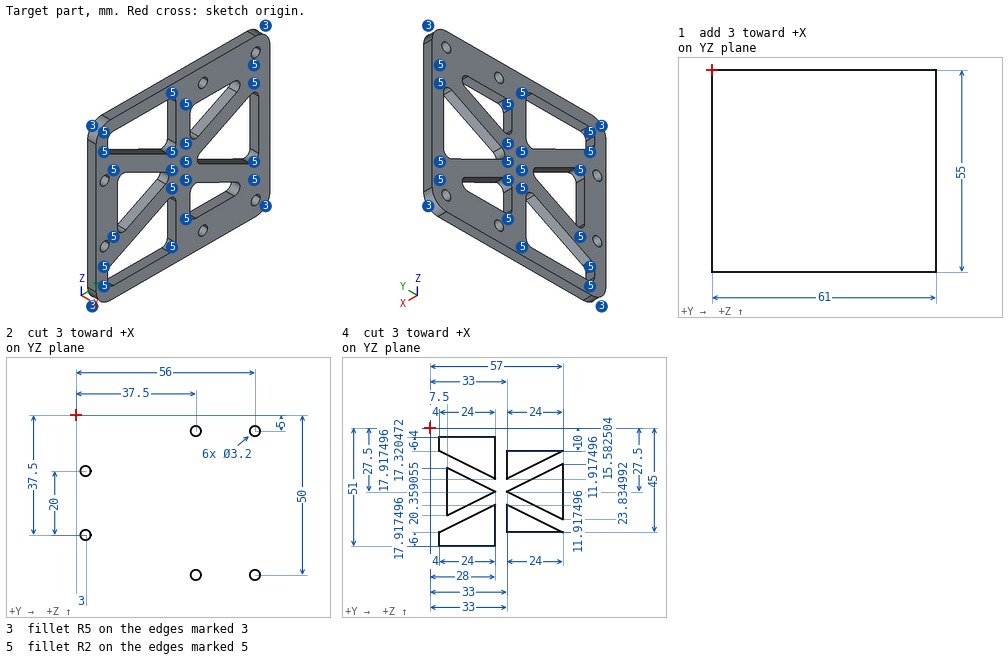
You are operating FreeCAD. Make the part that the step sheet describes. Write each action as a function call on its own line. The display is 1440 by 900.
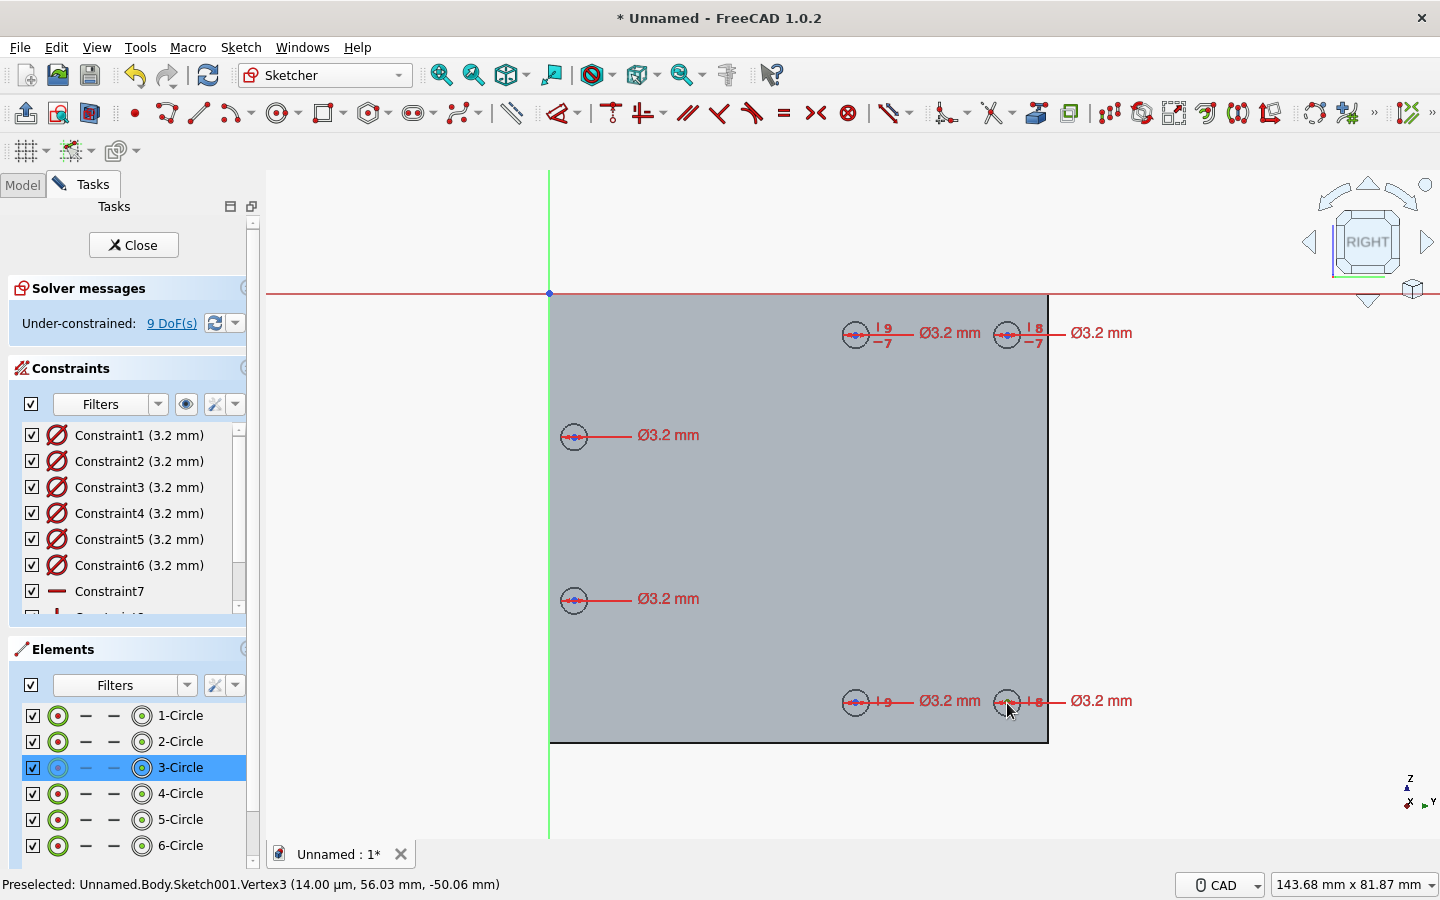
click(856, 703)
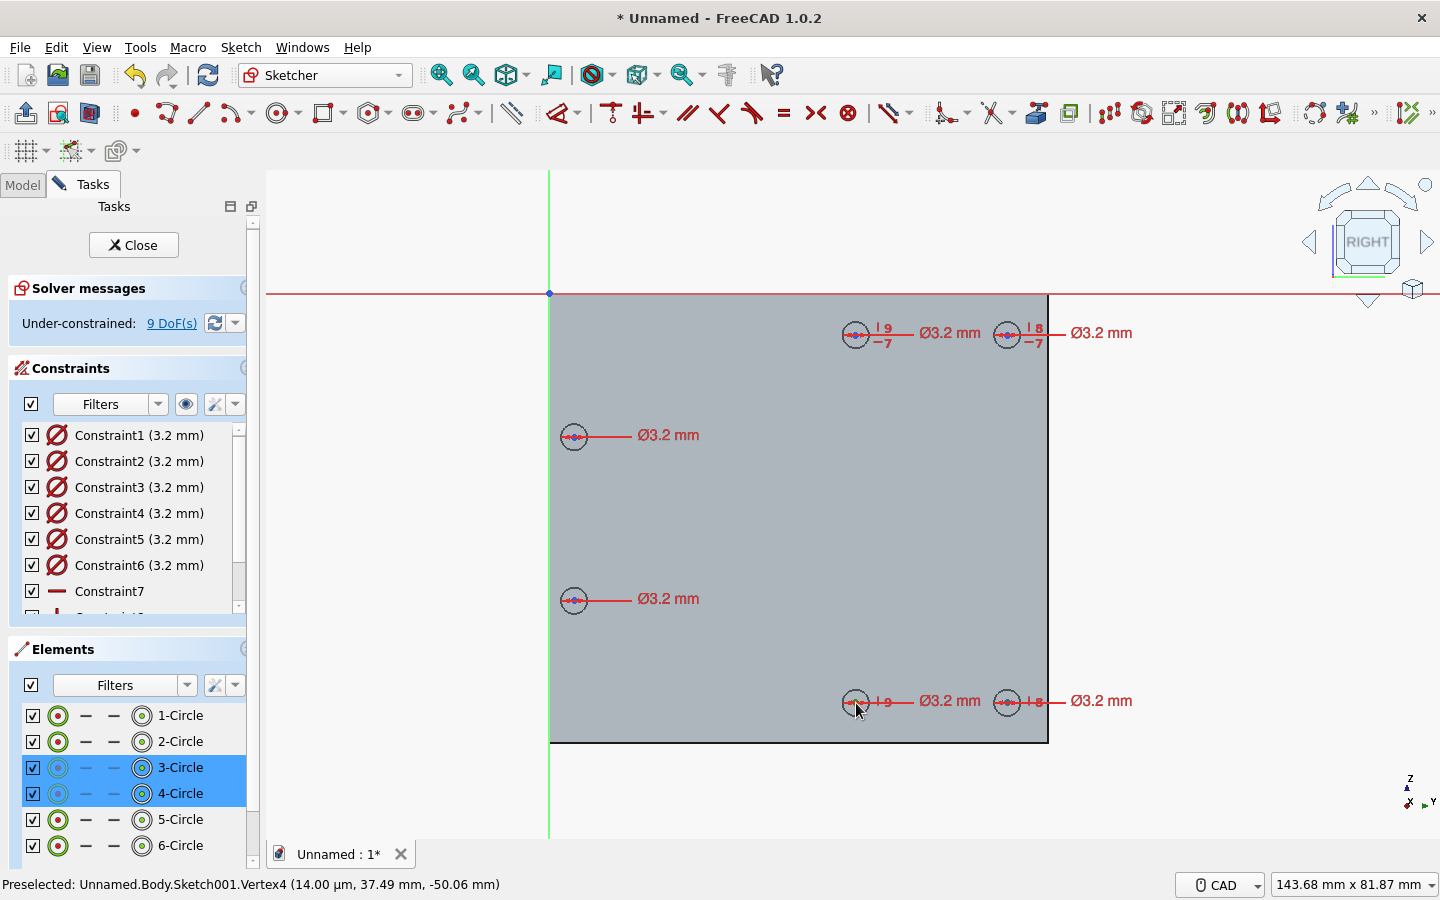
key(h)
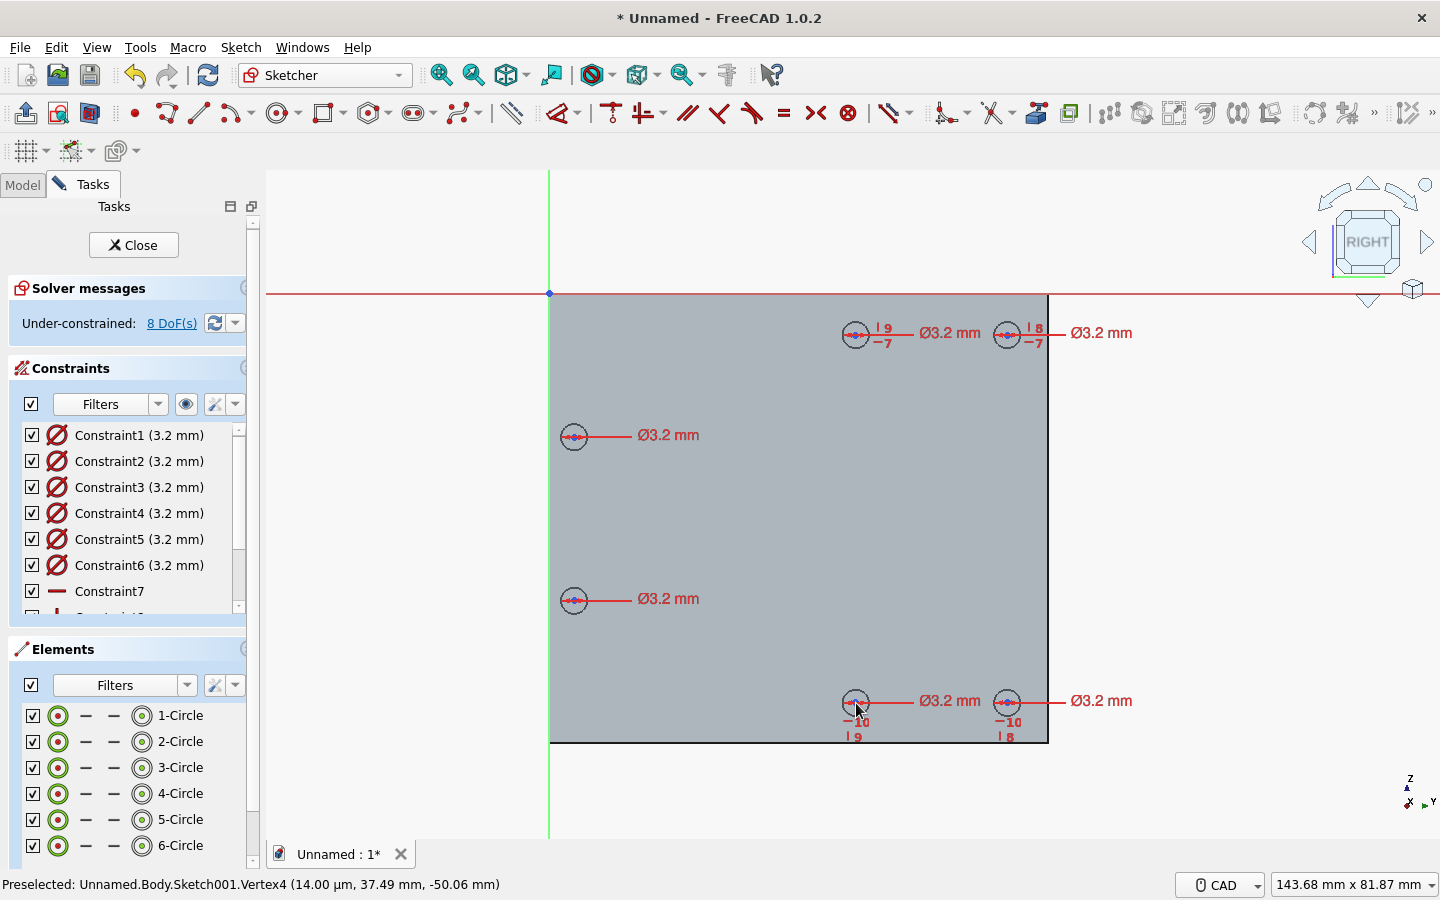
click(574, 601)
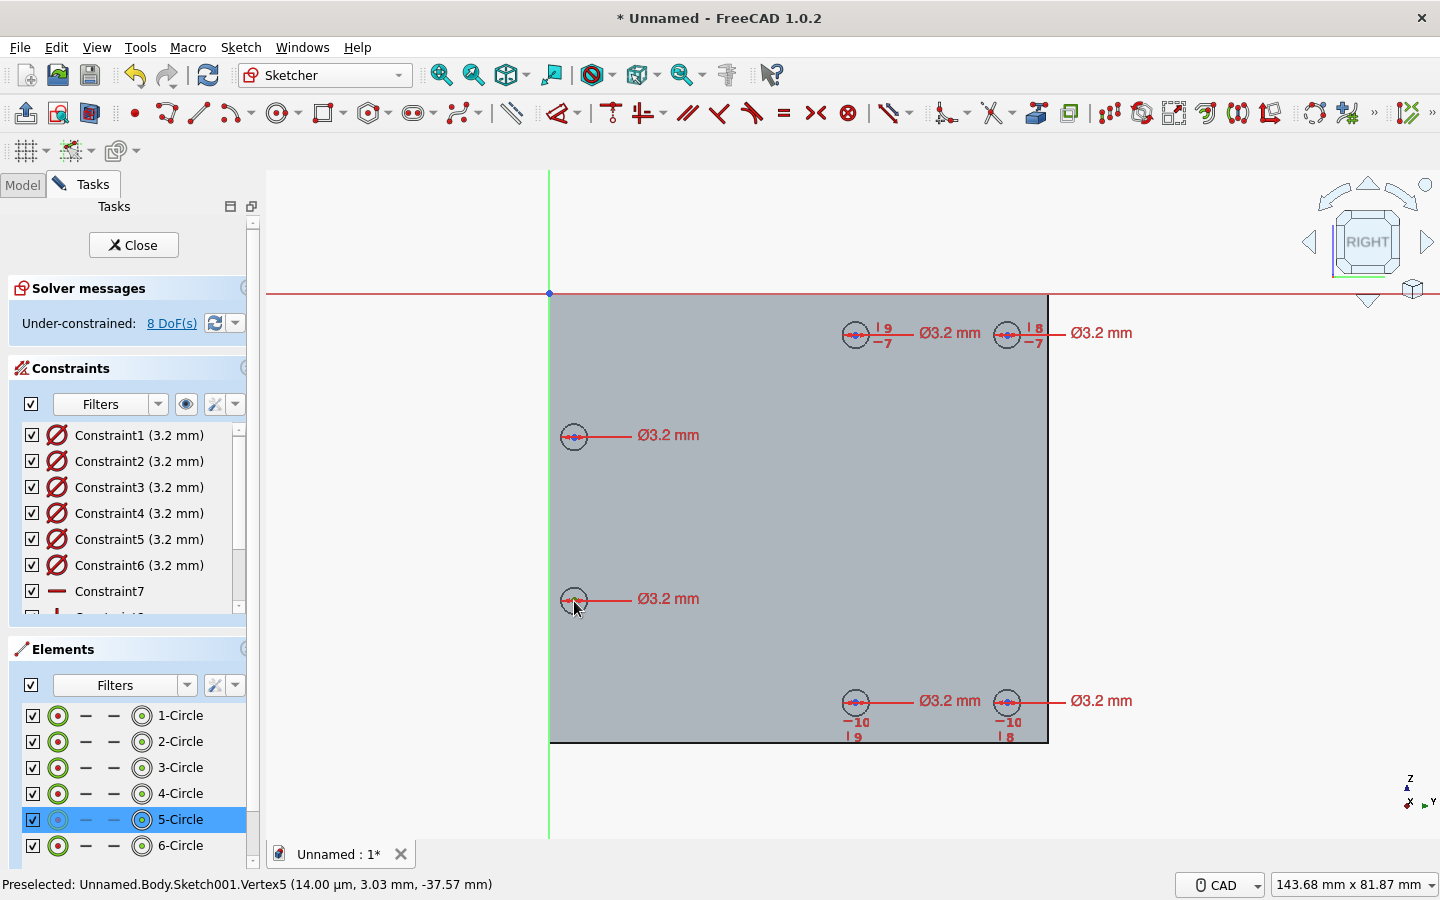
click(574, 437)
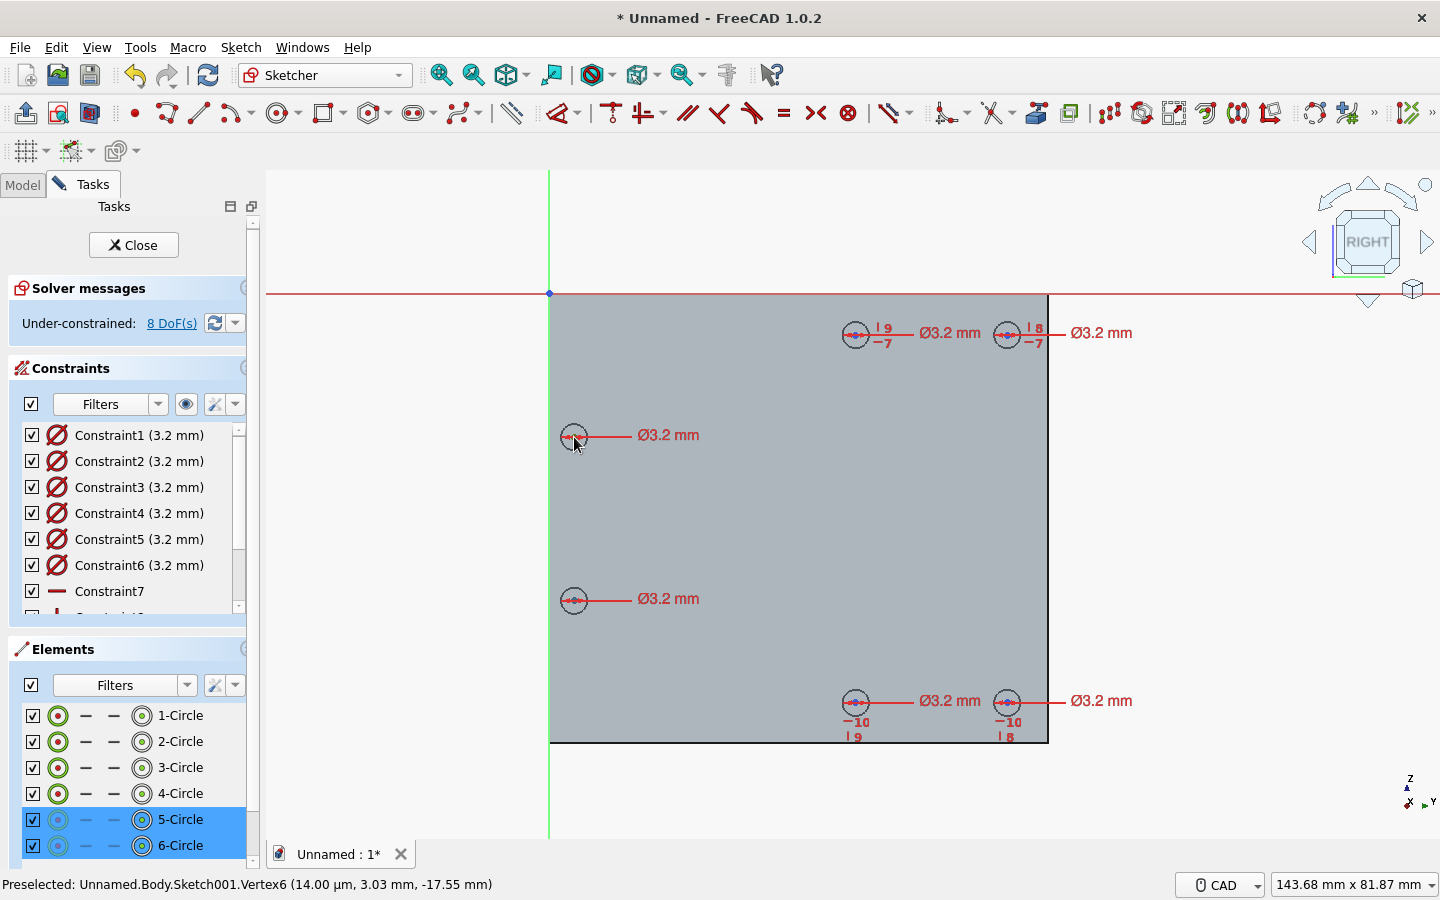
key(v)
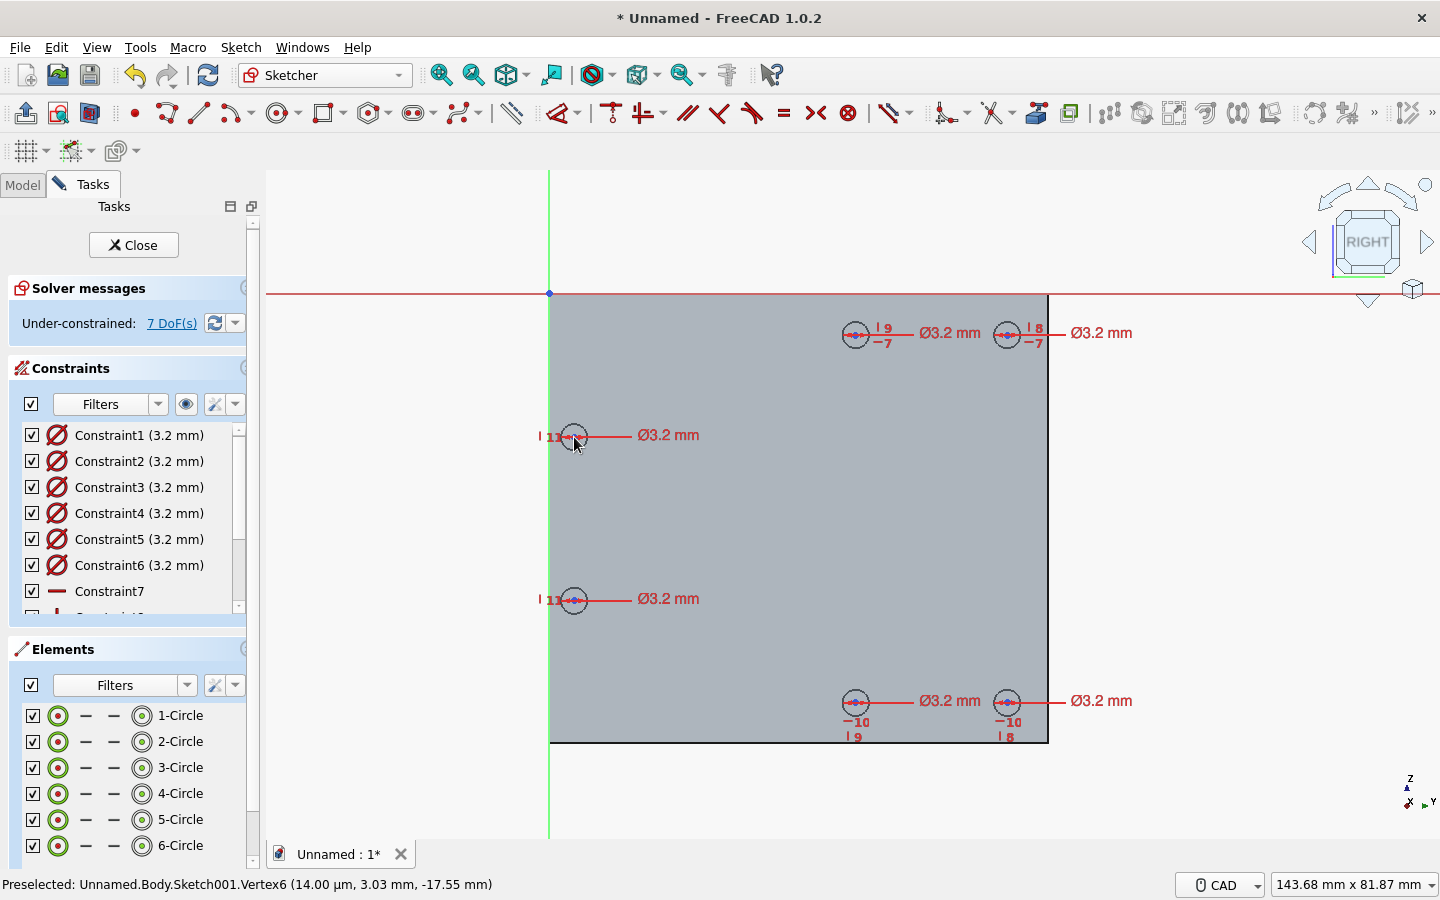
click(558, 114)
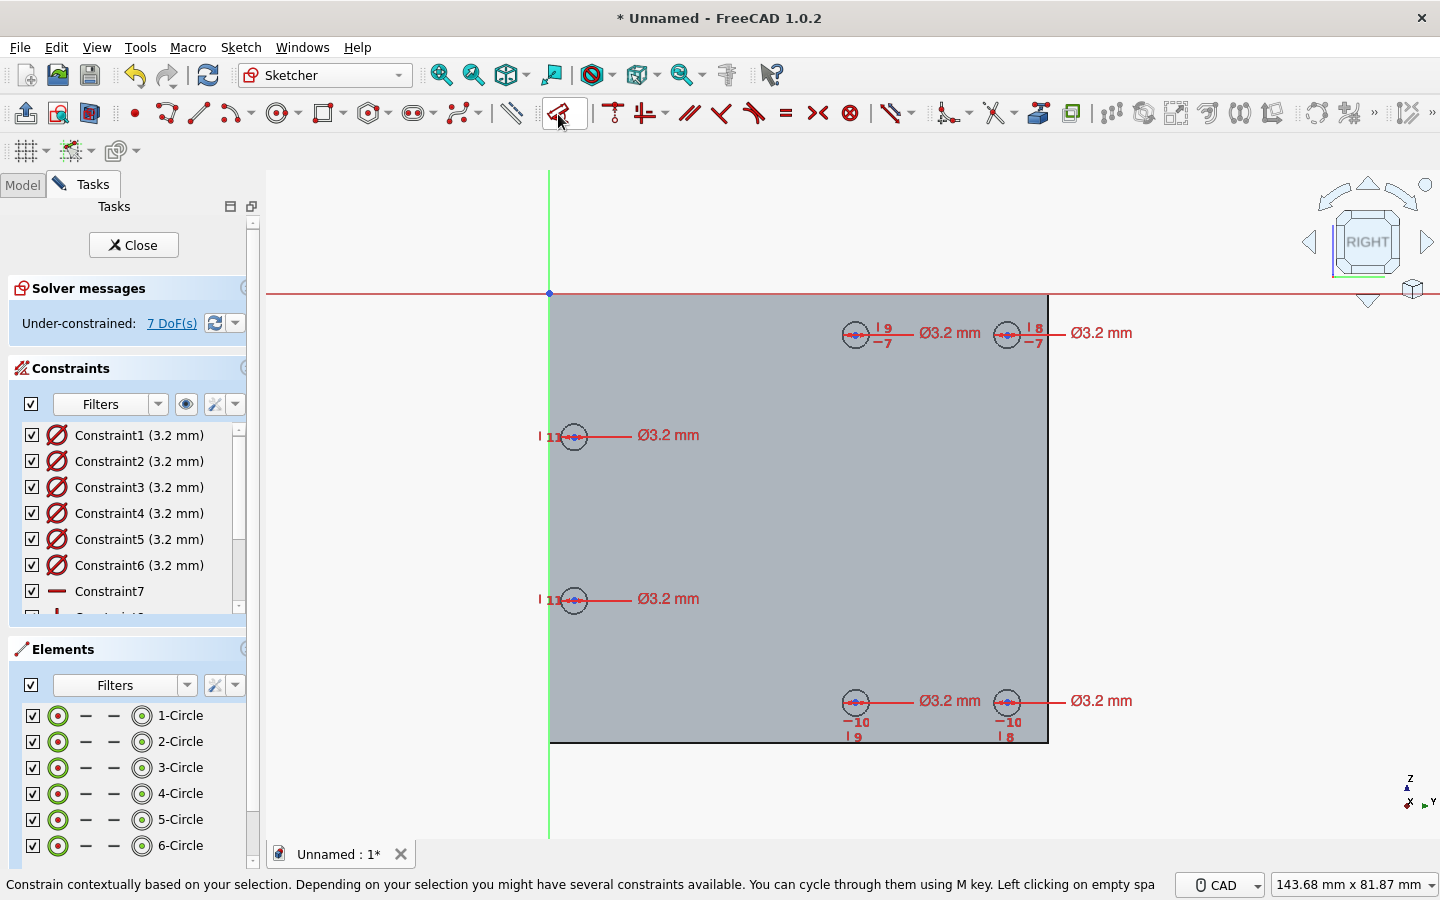
click(1007, 335)
click(515, 314)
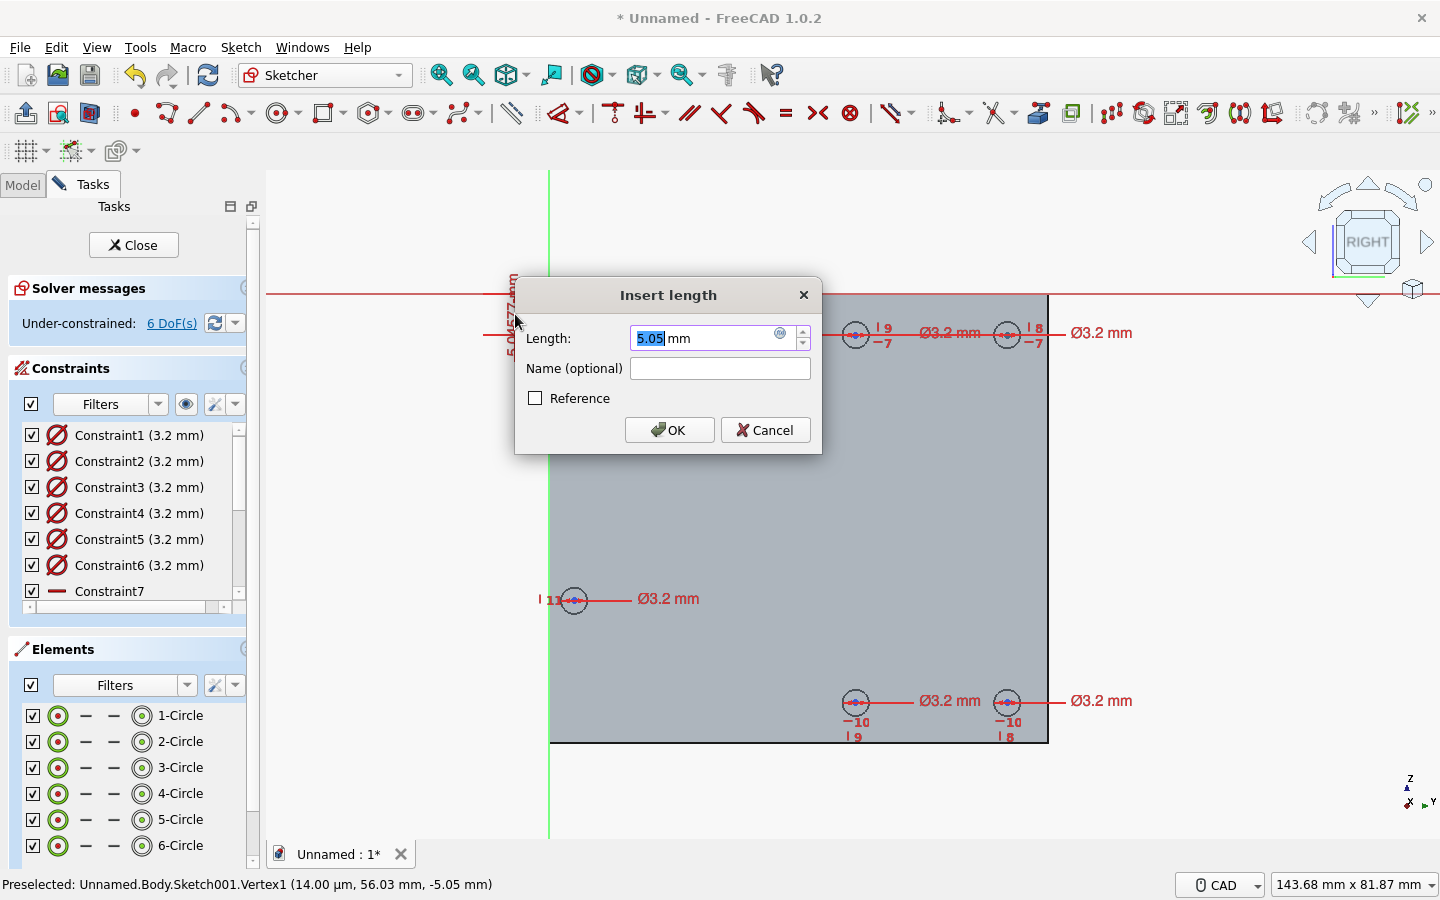
text(5)
key(Return)